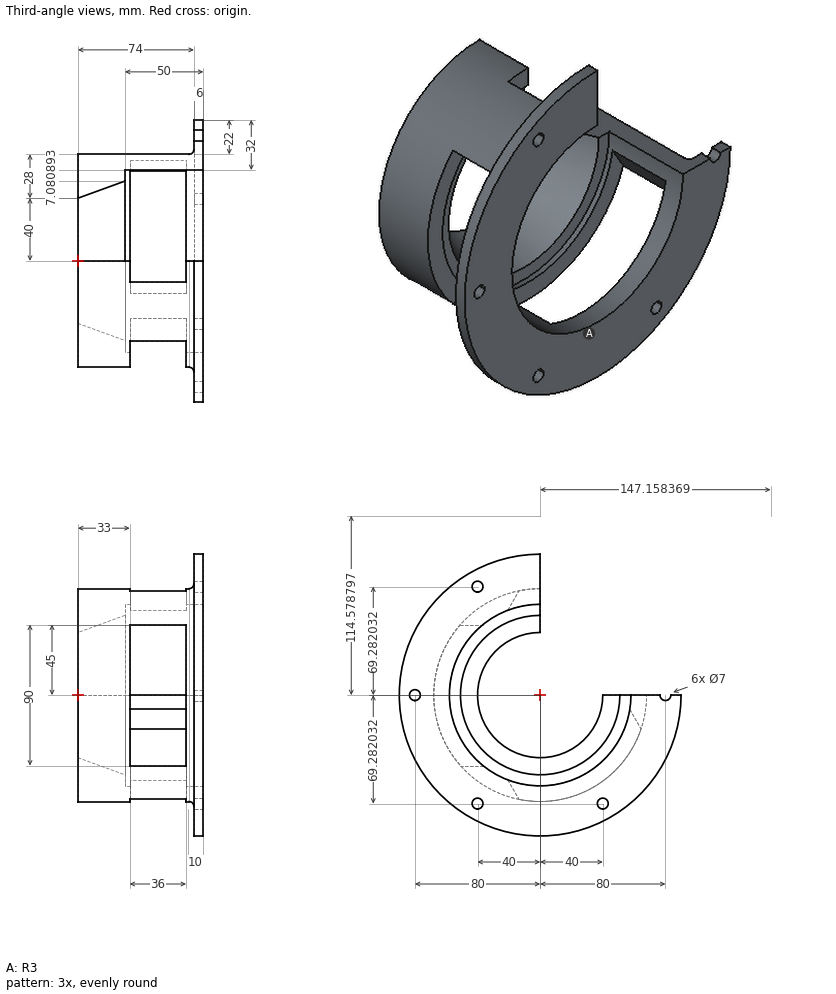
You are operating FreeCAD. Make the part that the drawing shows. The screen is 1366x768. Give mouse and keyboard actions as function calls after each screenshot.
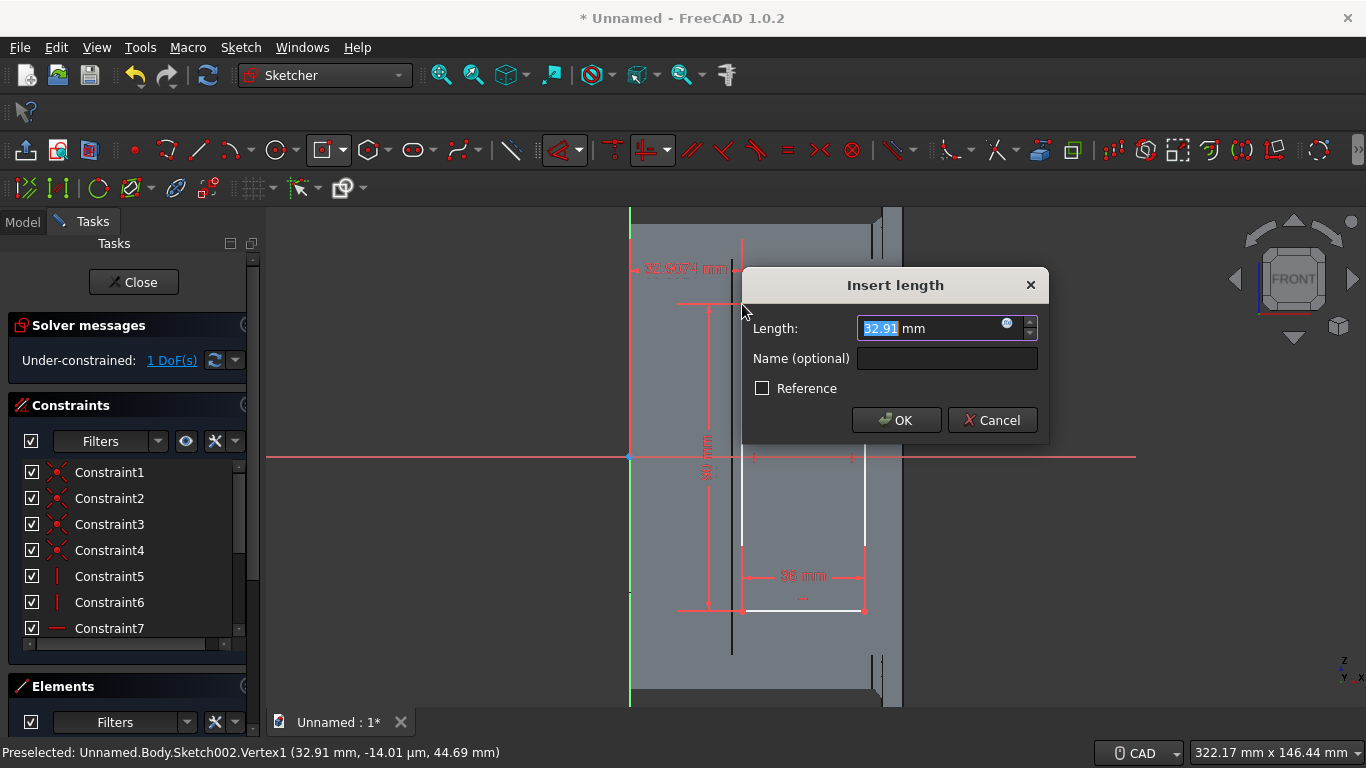
text(33)
key(Return)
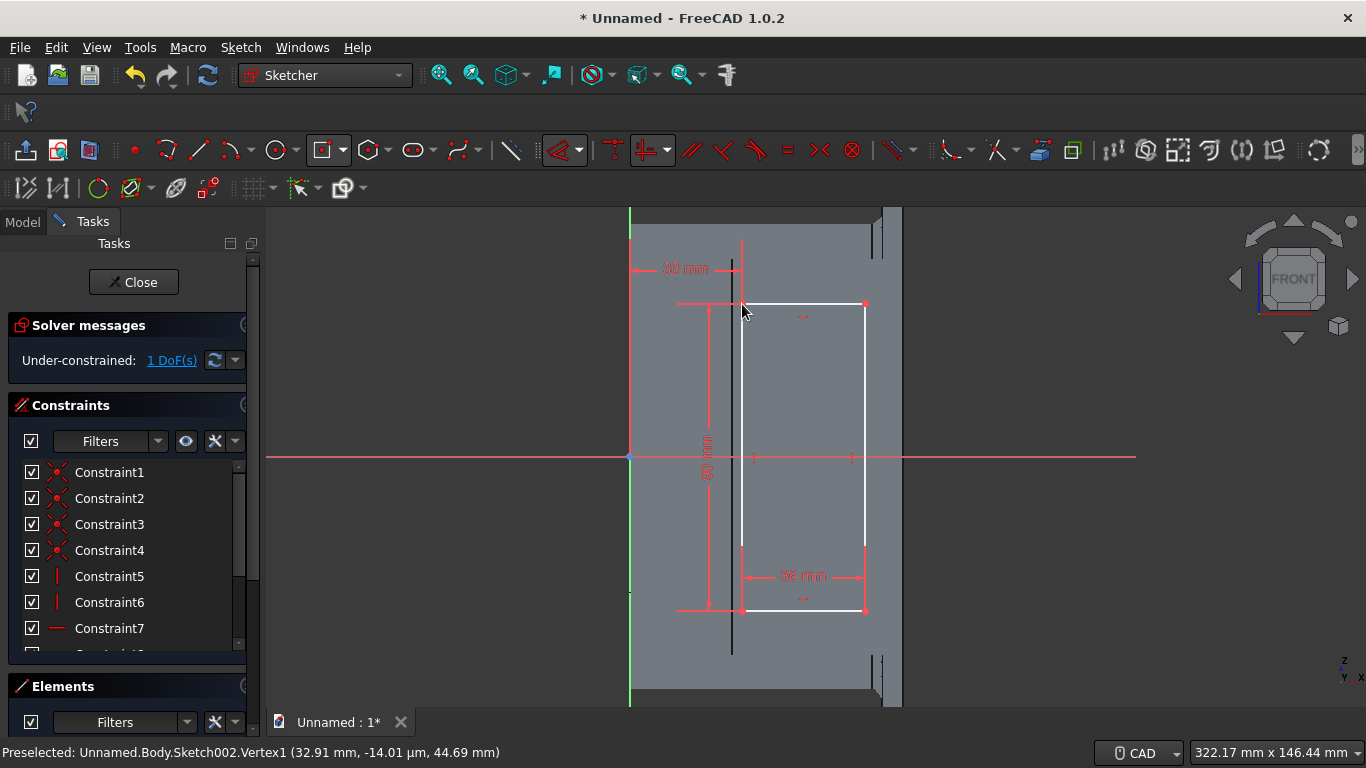
click(742, 304)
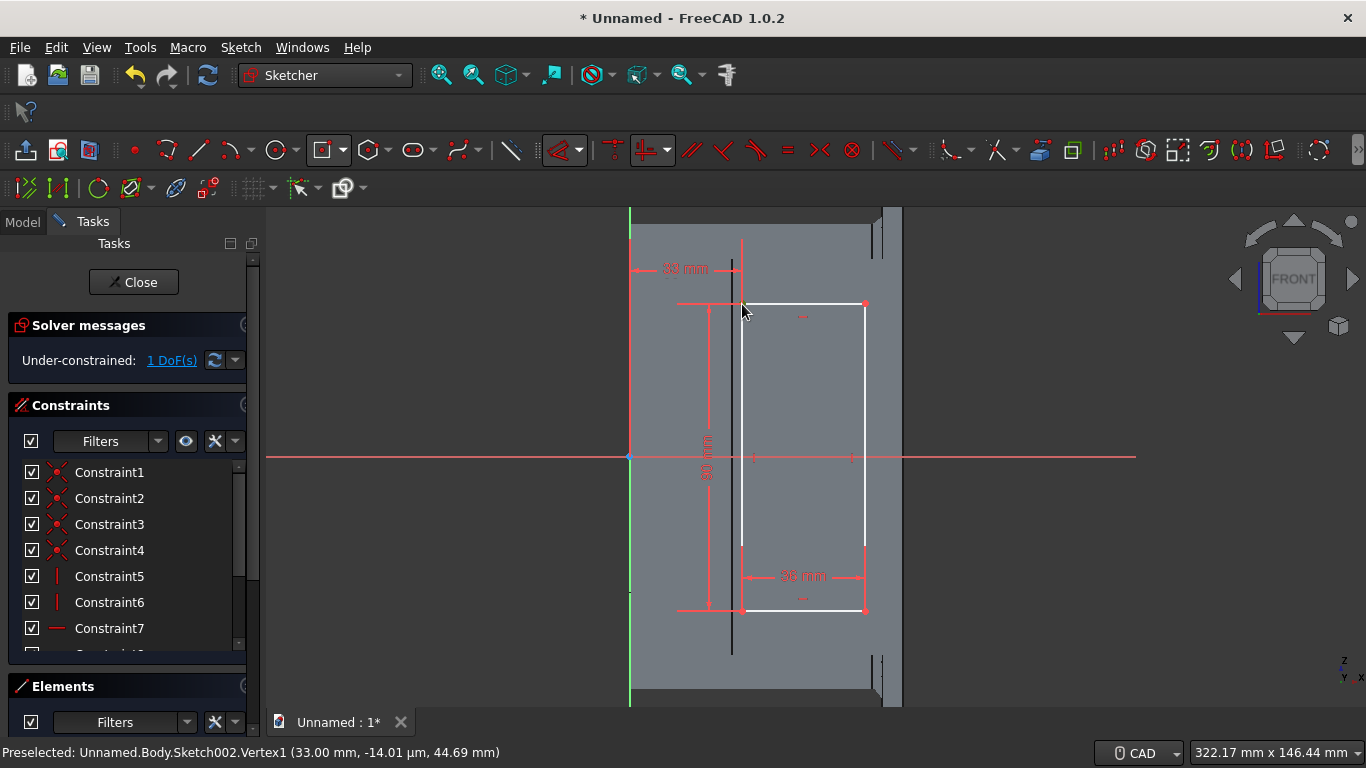
key(i)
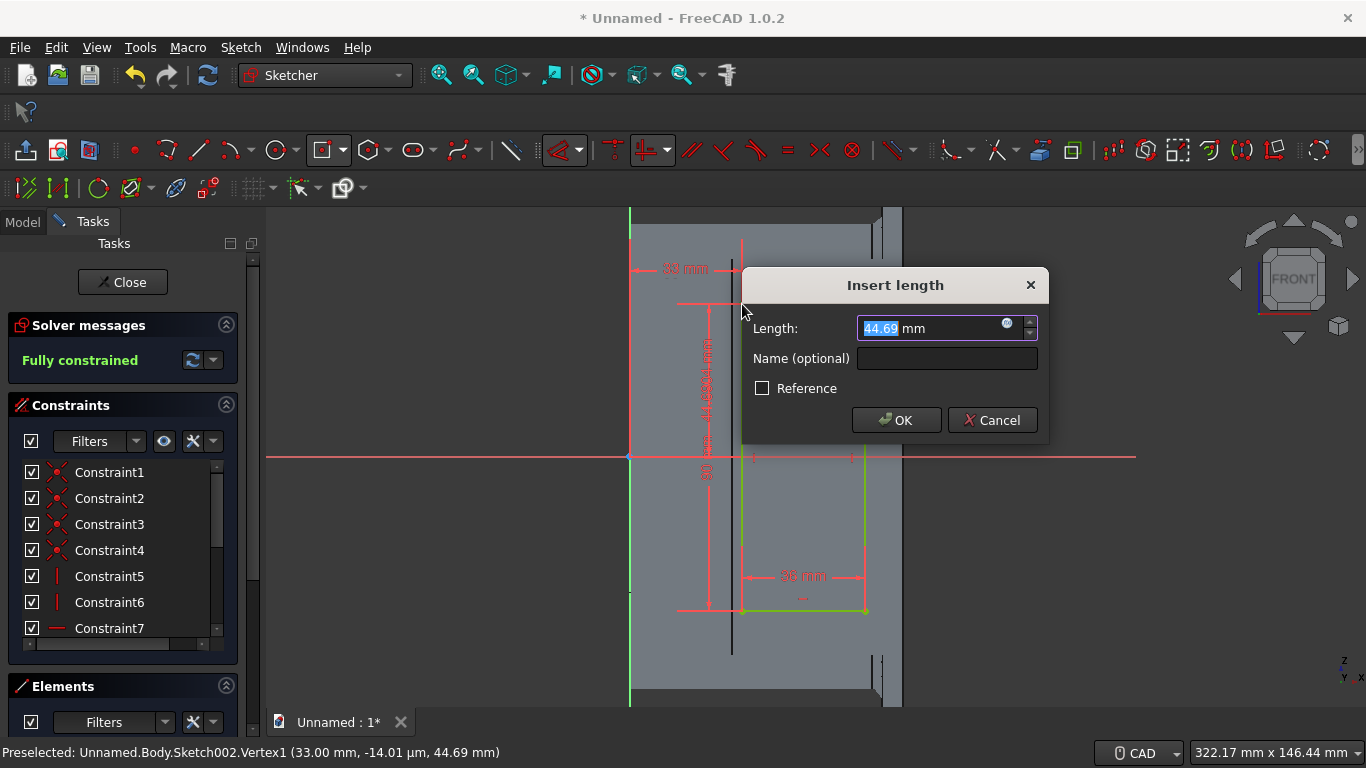
text(45)
key(Return)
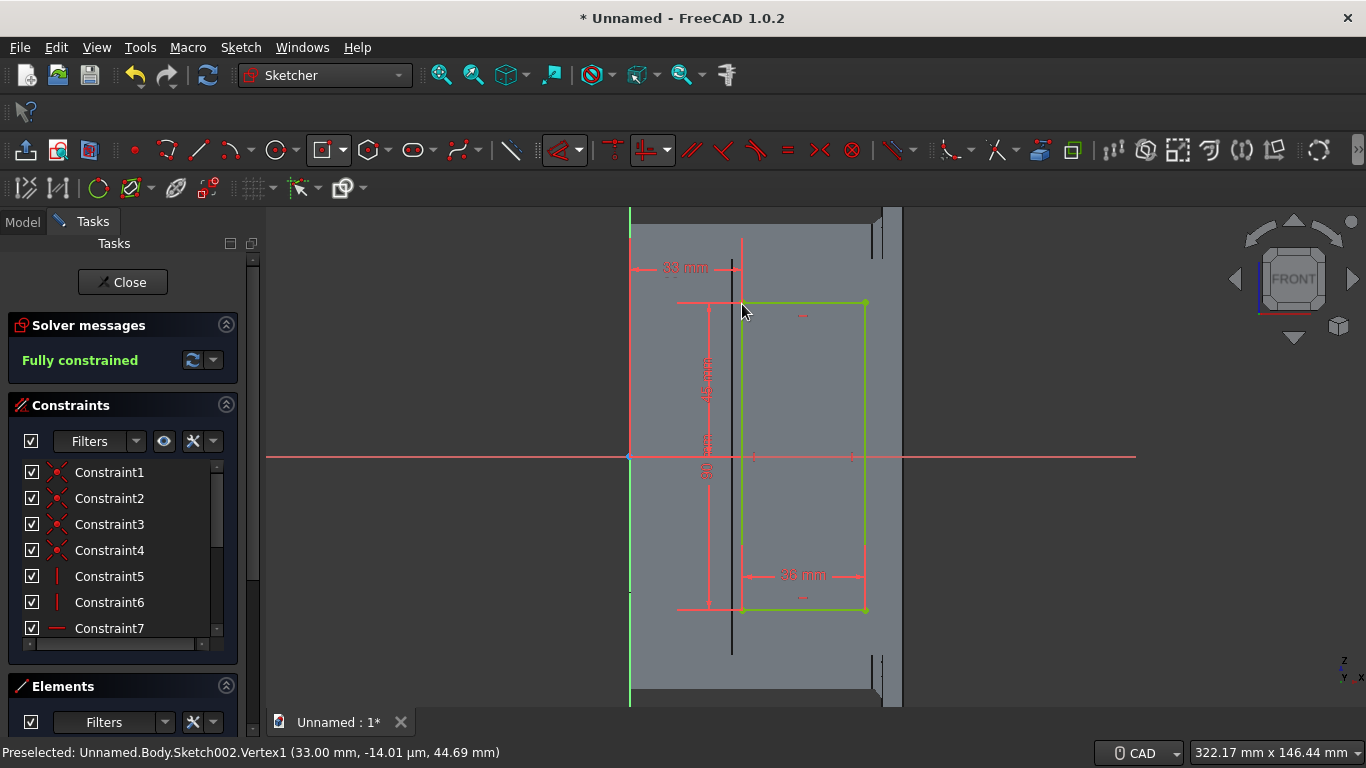
click(123, 282)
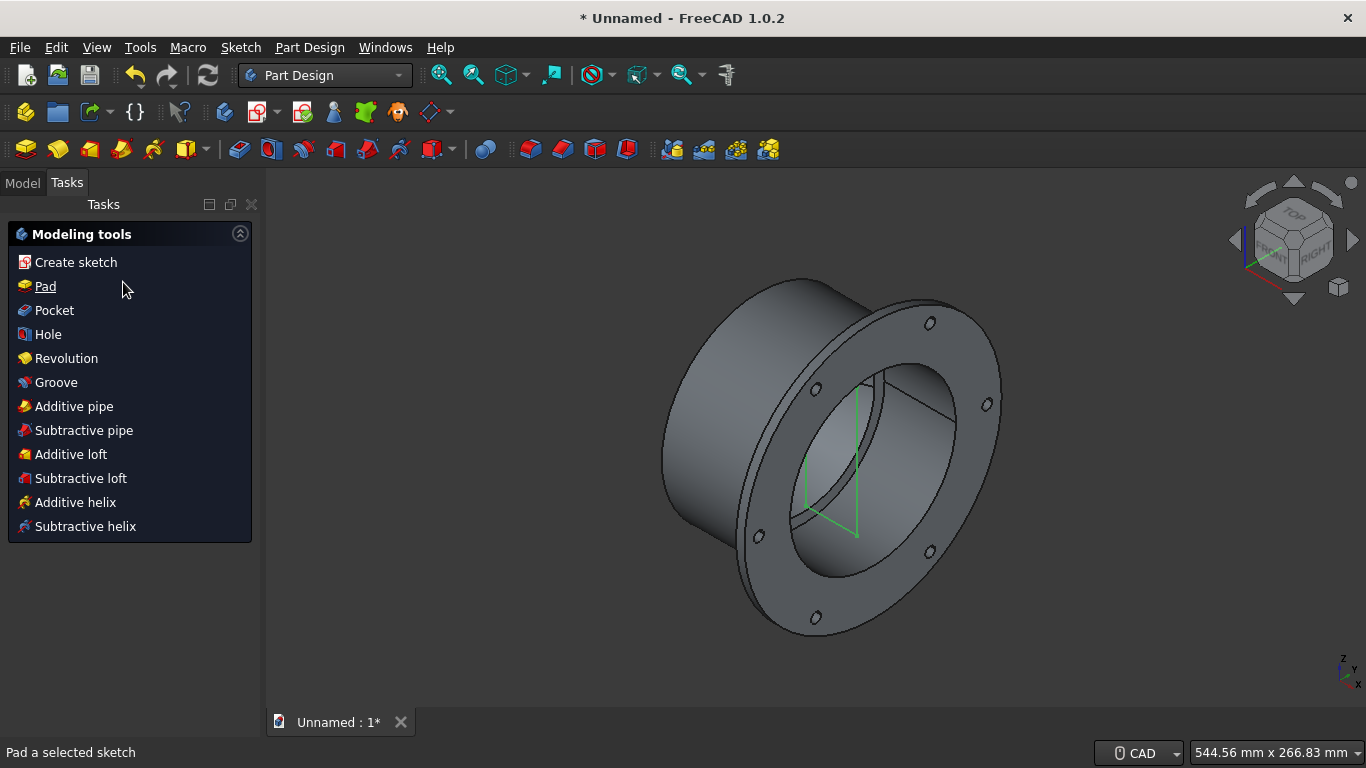
click(240, 150)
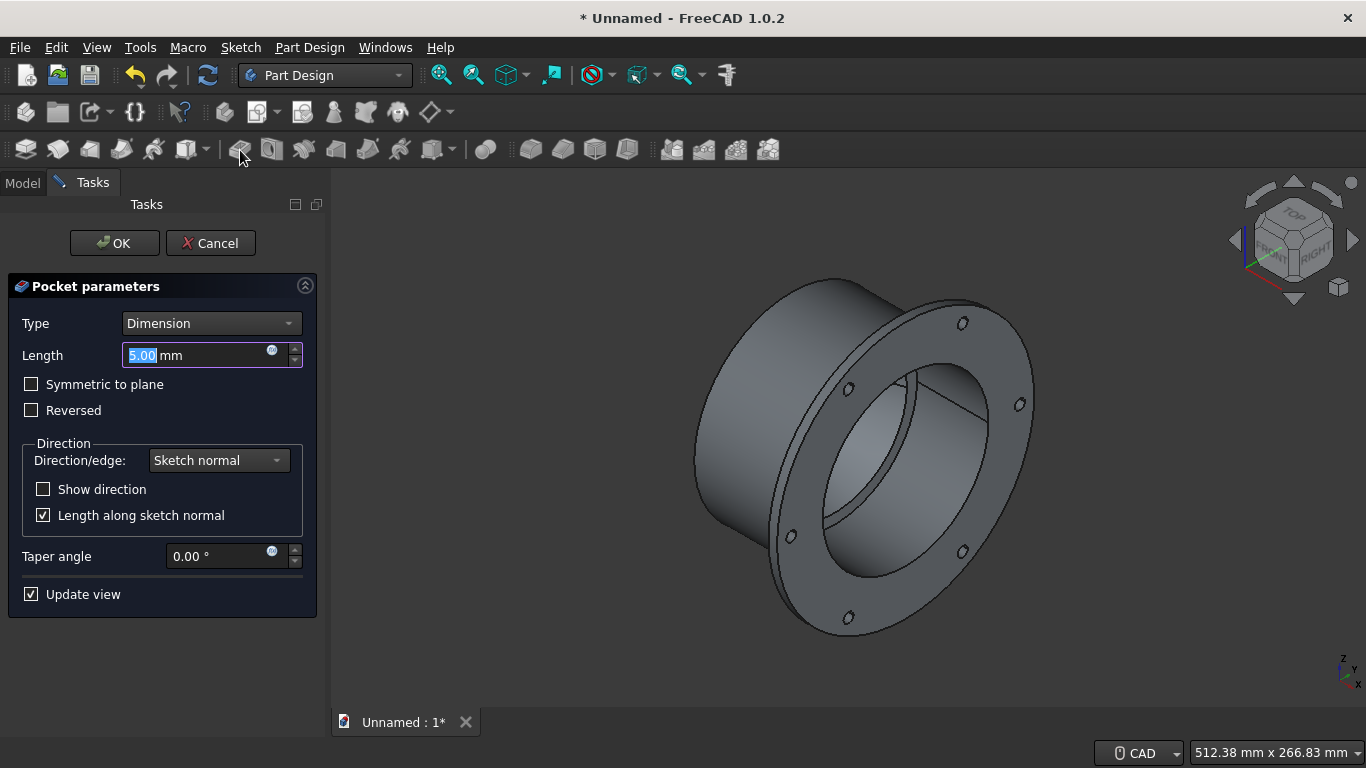
click(212, 324)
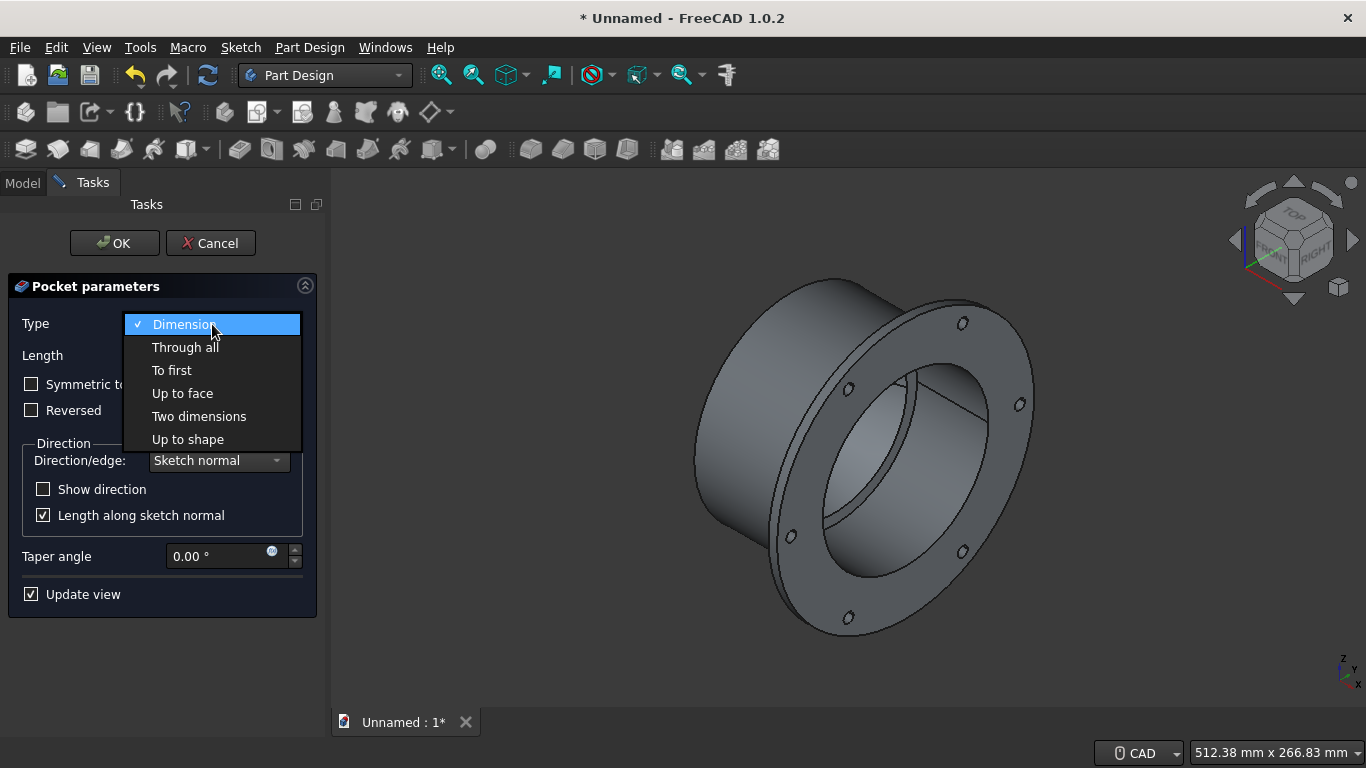
click(212, 348)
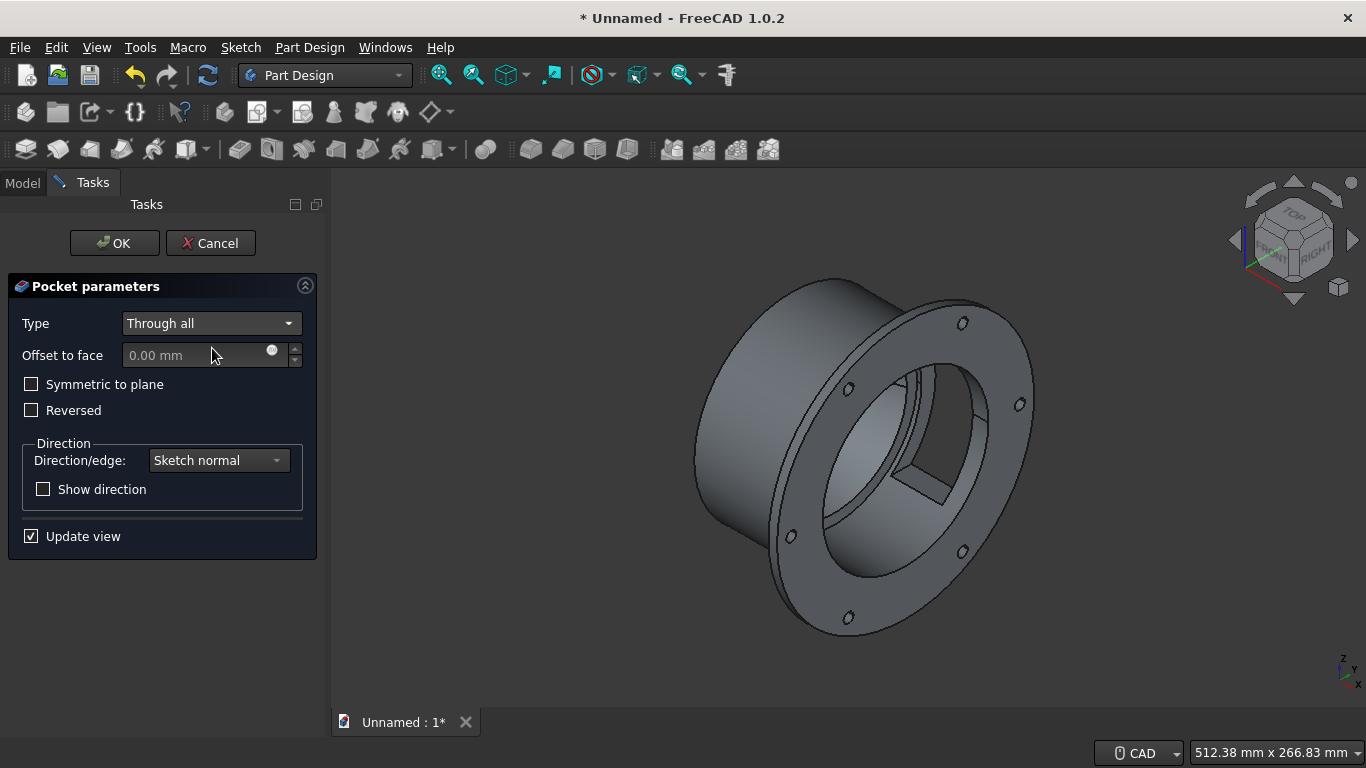
click(30, 410)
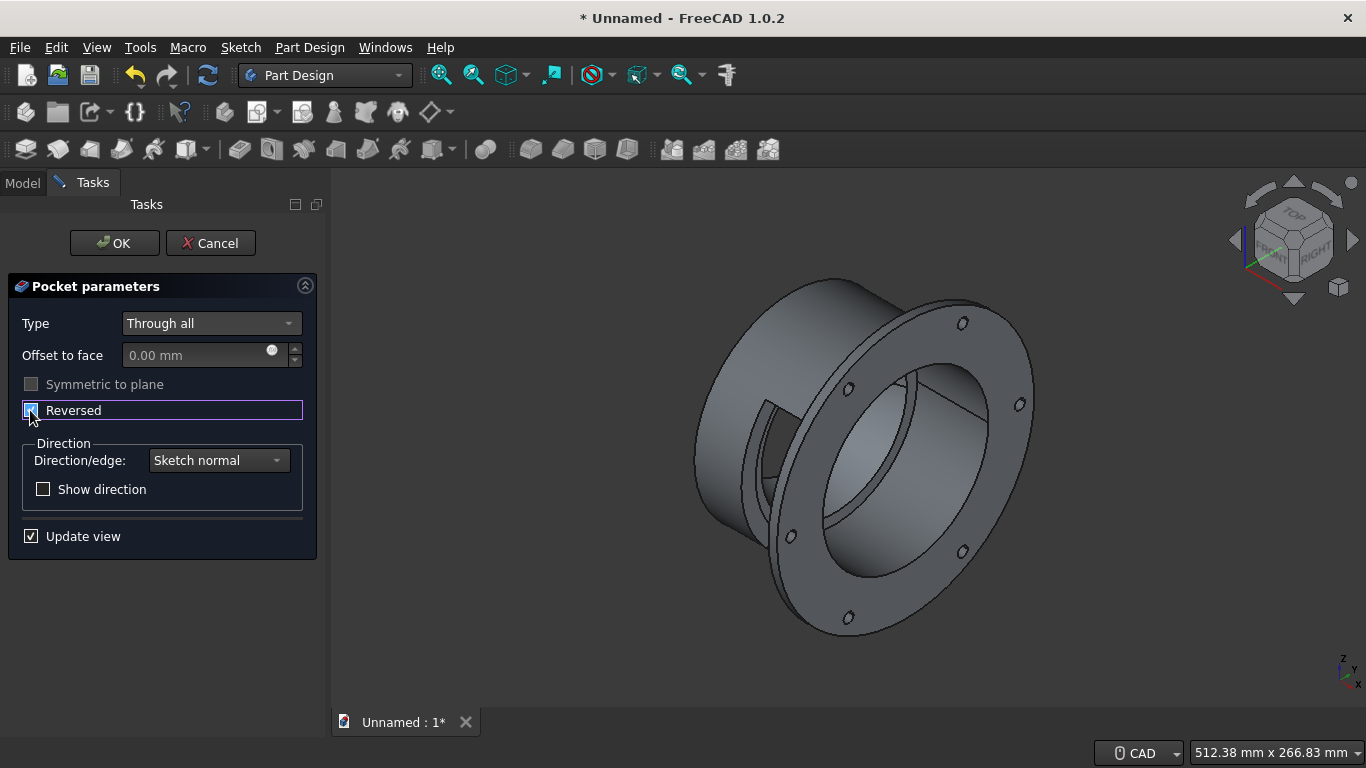
click(115, 243)